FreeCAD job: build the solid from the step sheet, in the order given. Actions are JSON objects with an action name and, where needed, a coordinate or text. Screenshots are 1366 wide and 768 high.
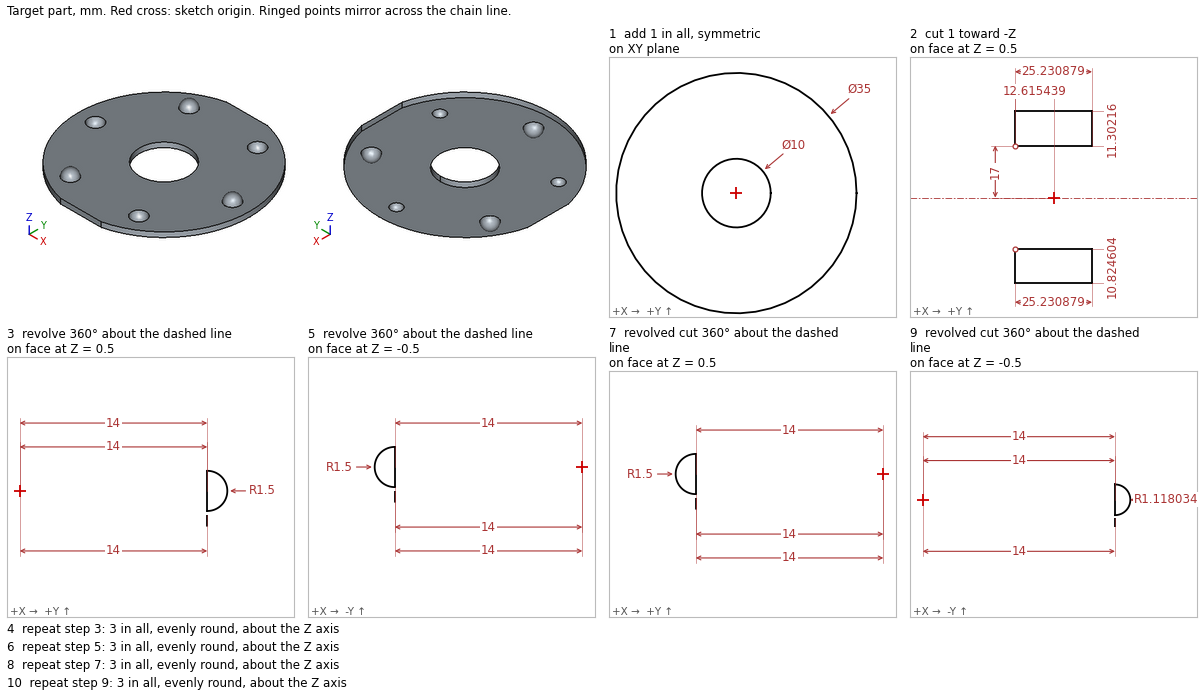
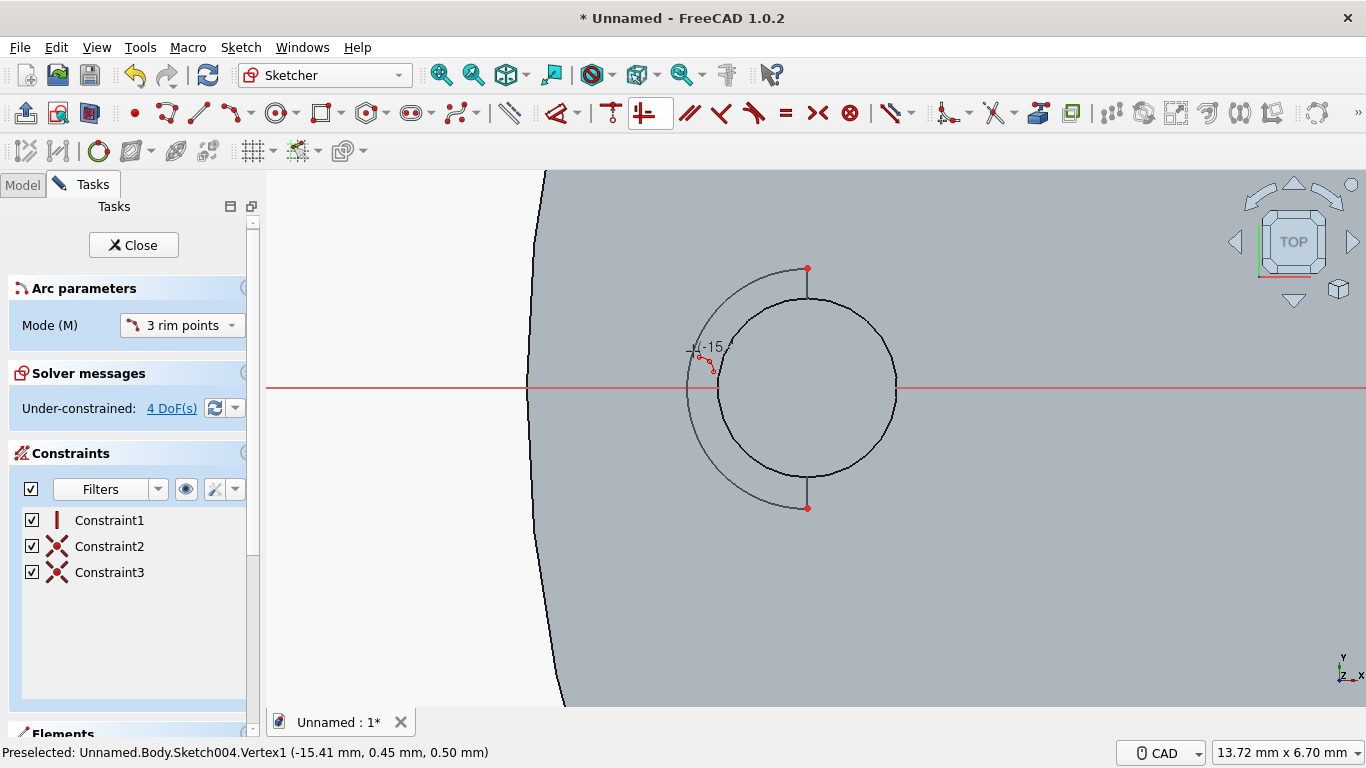
{"action": "key", "text": "g l"}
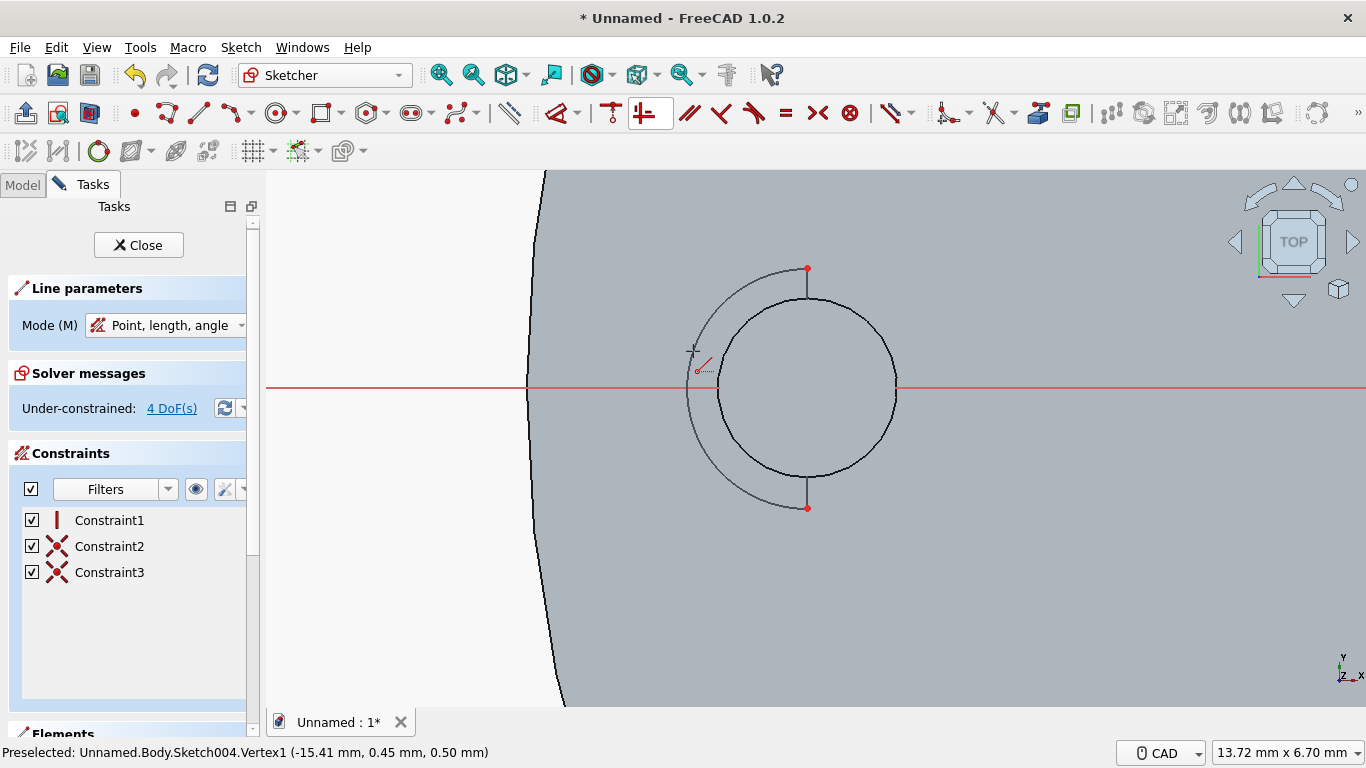
{"action": "left_click", "coordinate": [807, 532]}
{"action": "left_click", "coordinate": [807, 604]}
{"action": "key", "text": "Escape"}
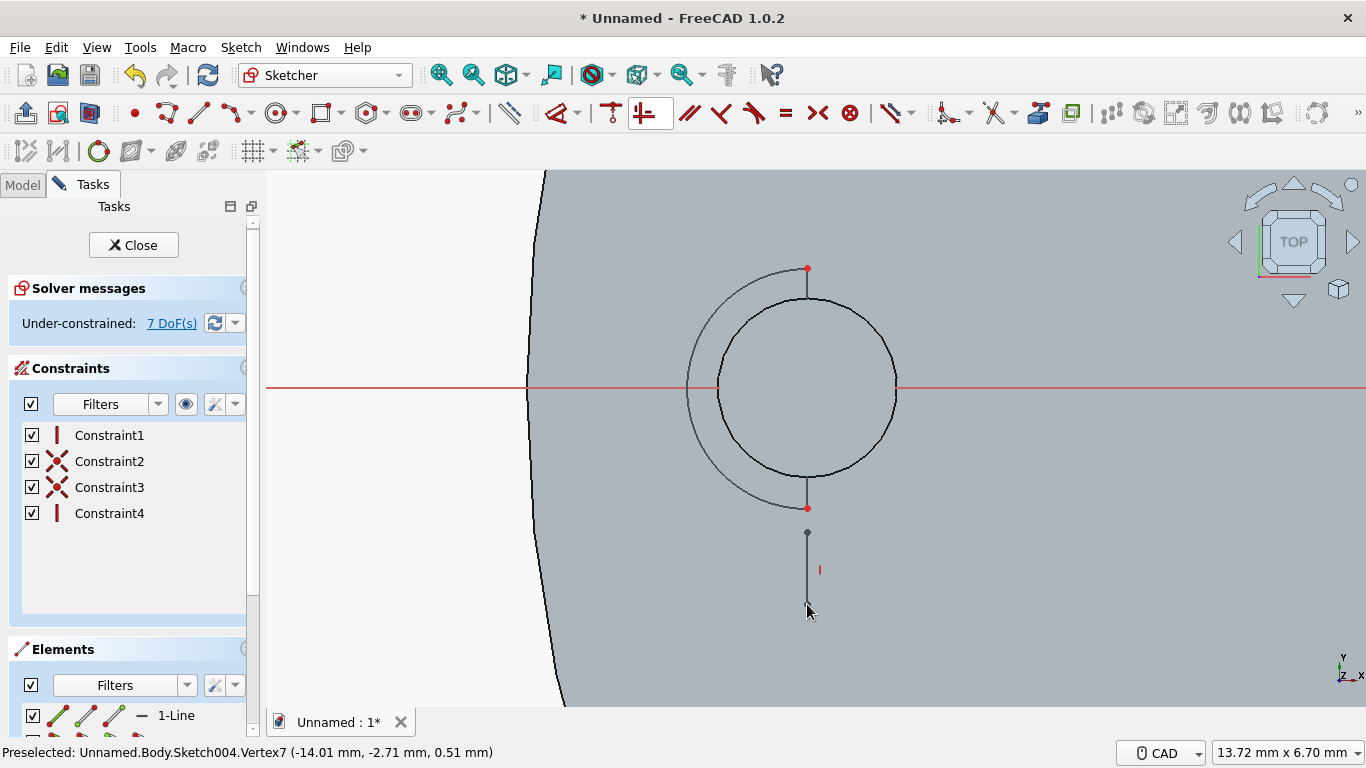
{"action": "left_click", "coordinate": [807, 555]}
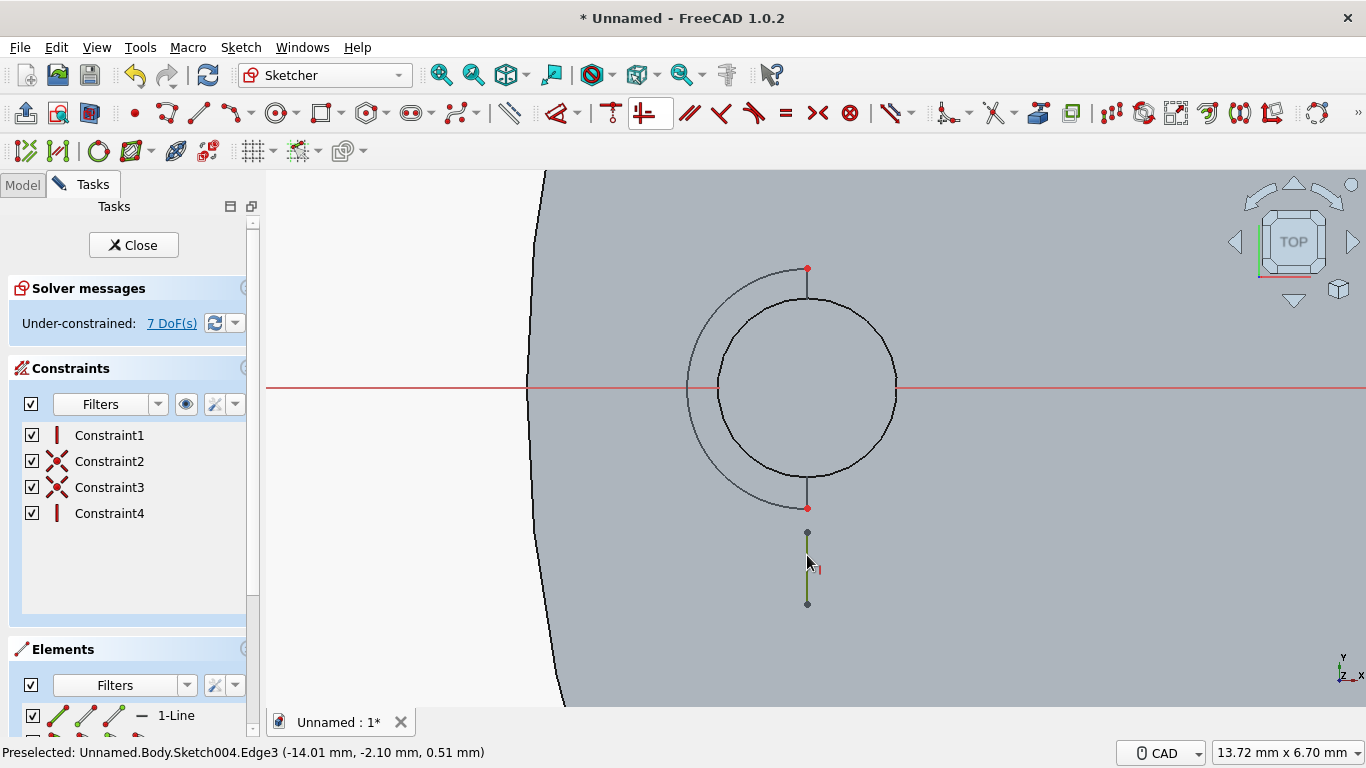
{"action": "key", "text": "g n"}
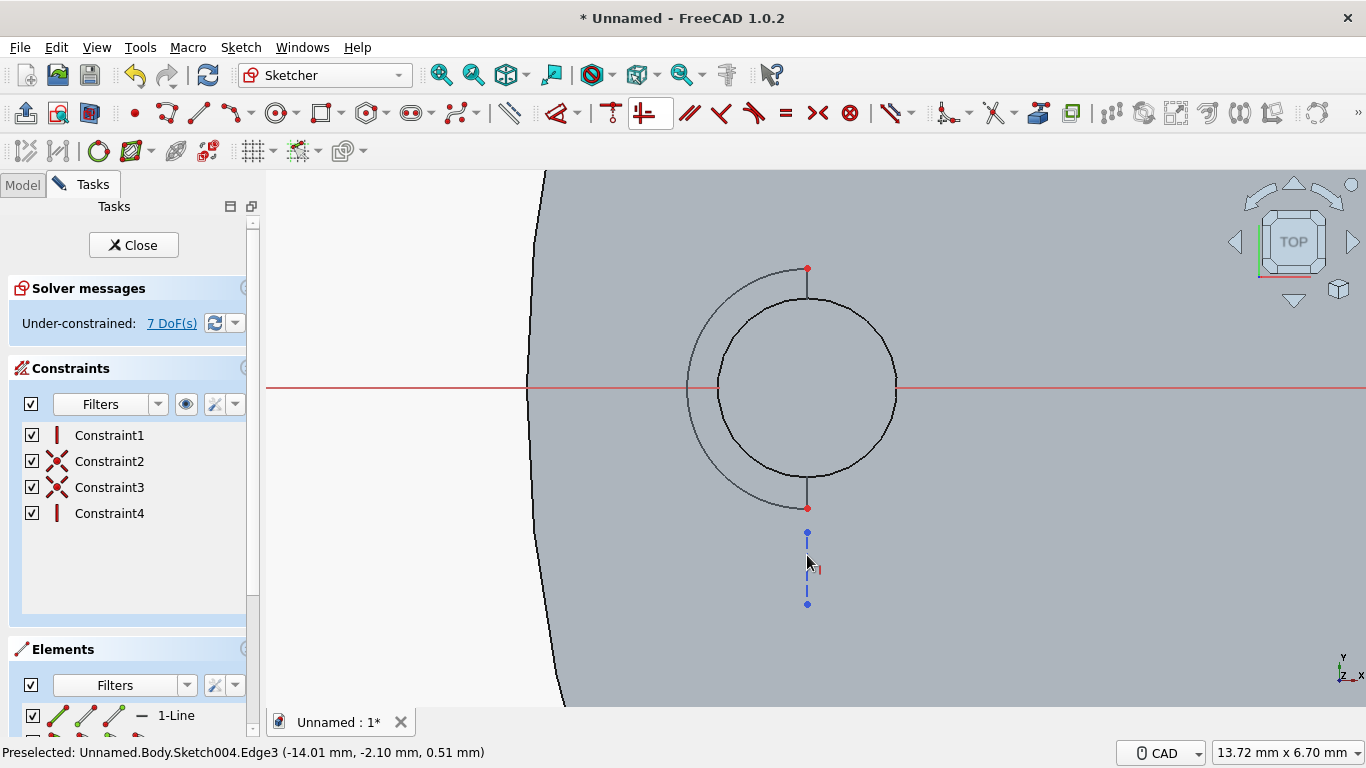
{"action": "left_click", "coordinate": [807, 389]}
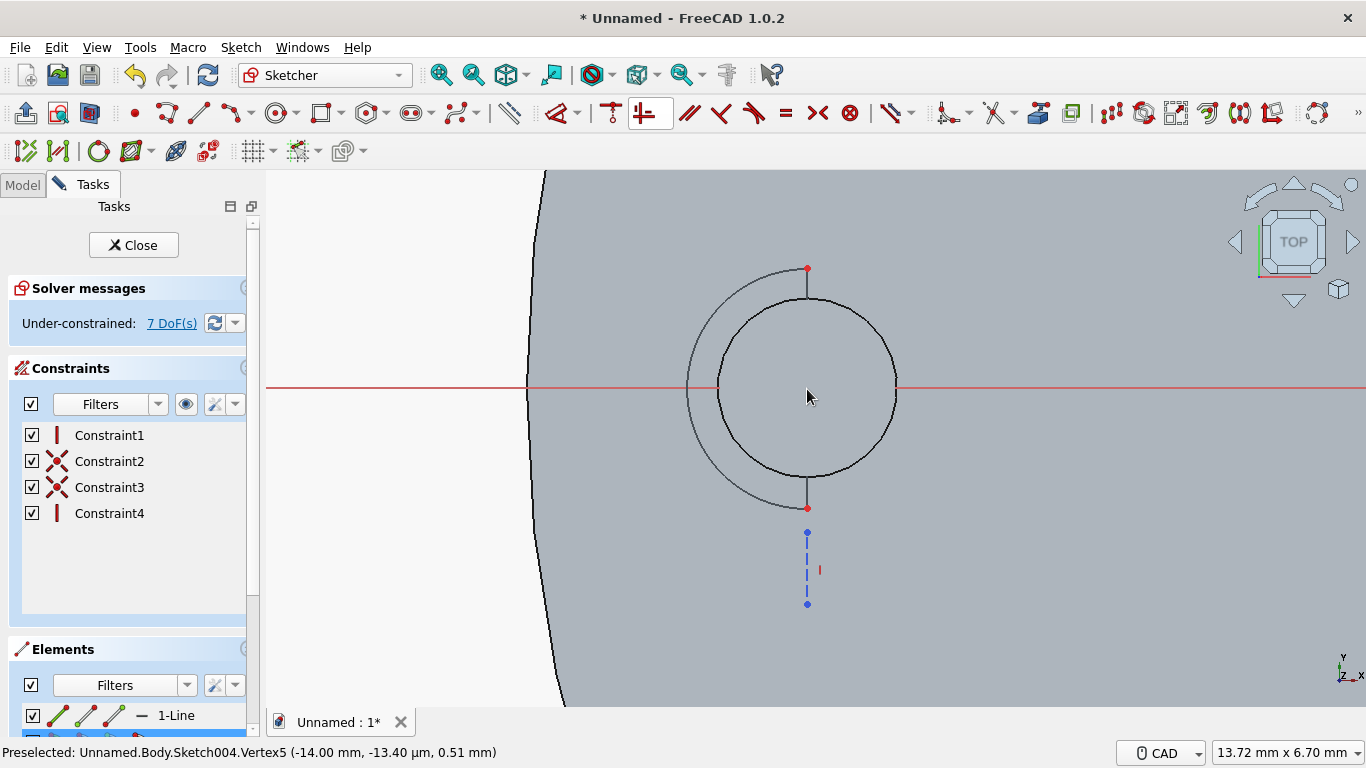
{"action": "left_click", "coordinate": [359, 388]}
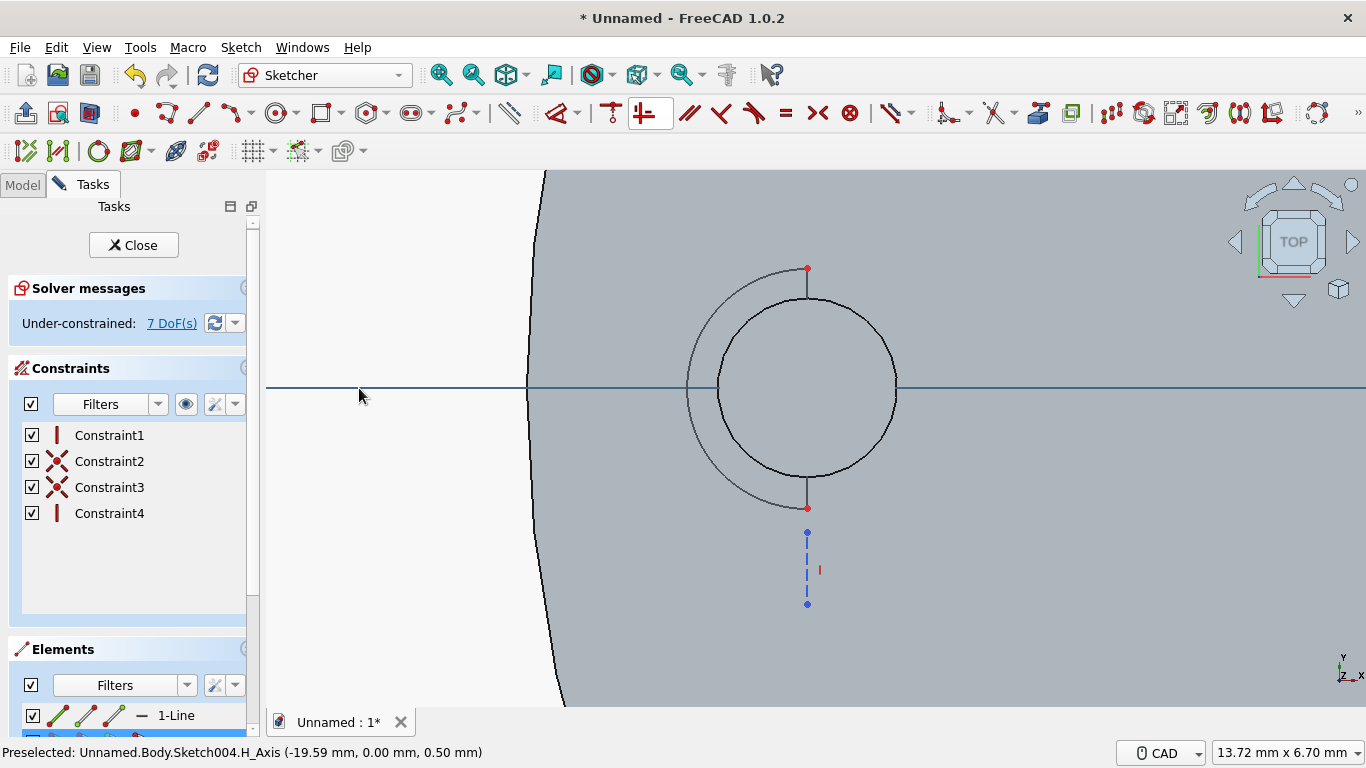
{"action": "left_click", "coordinate": [612, 114]}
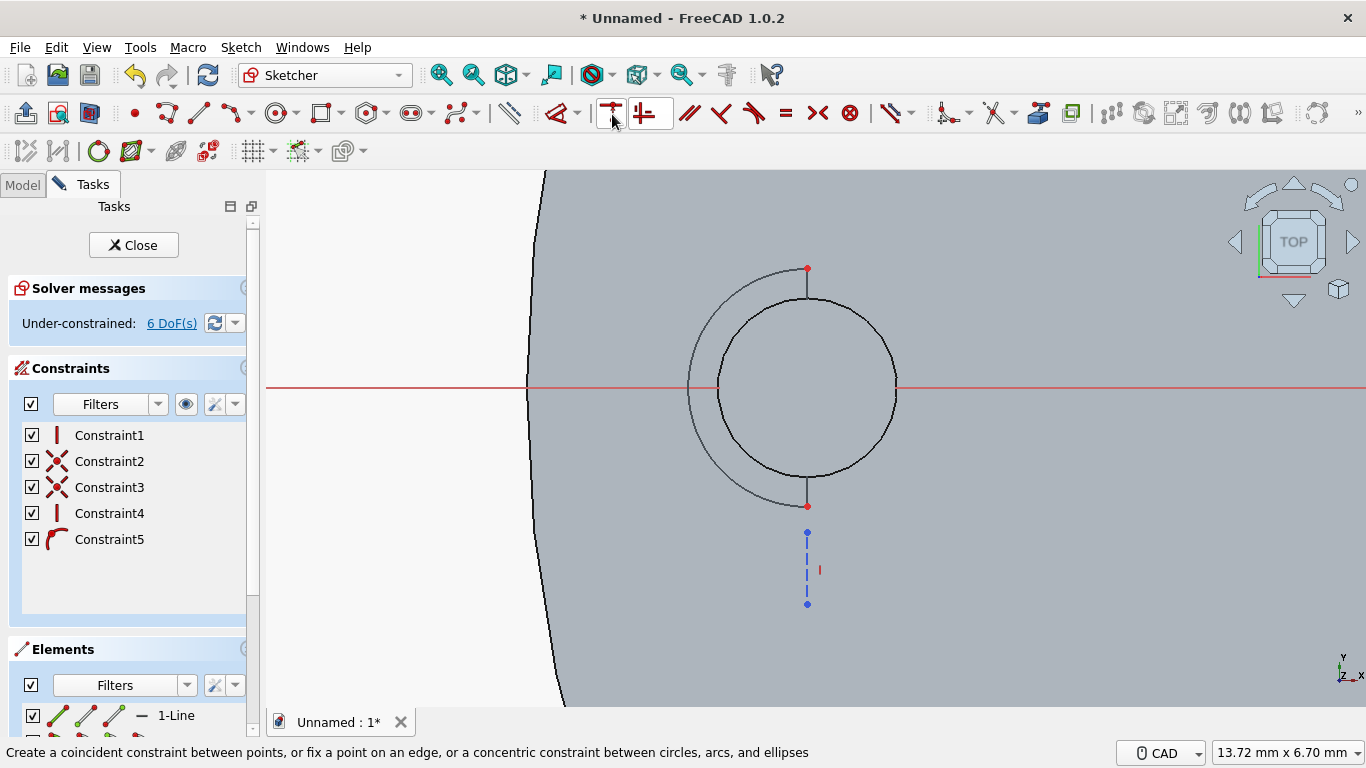
{"action": "key", "text": "d"}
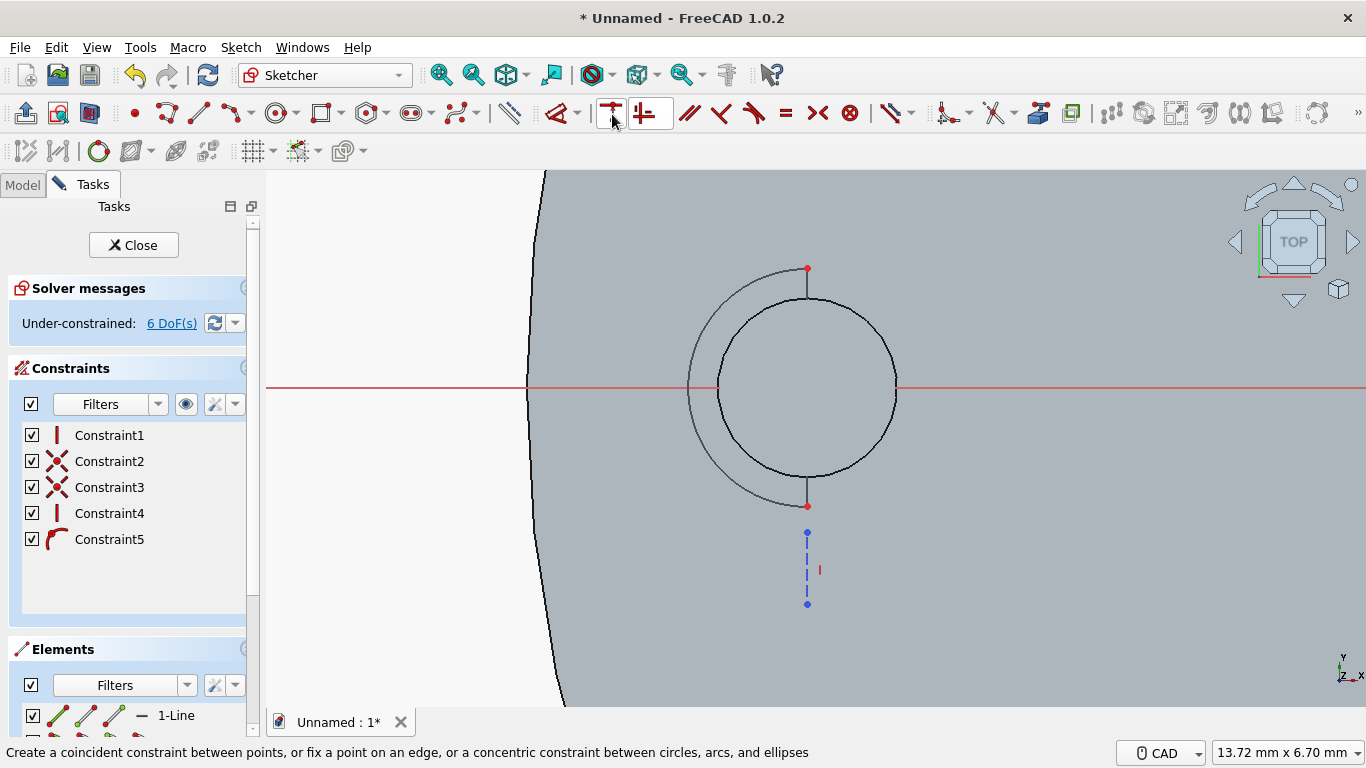
{"action": "left_click", "coordinate": [711, 318]}
{"action": "left_click", "coordinate": [685, 299]}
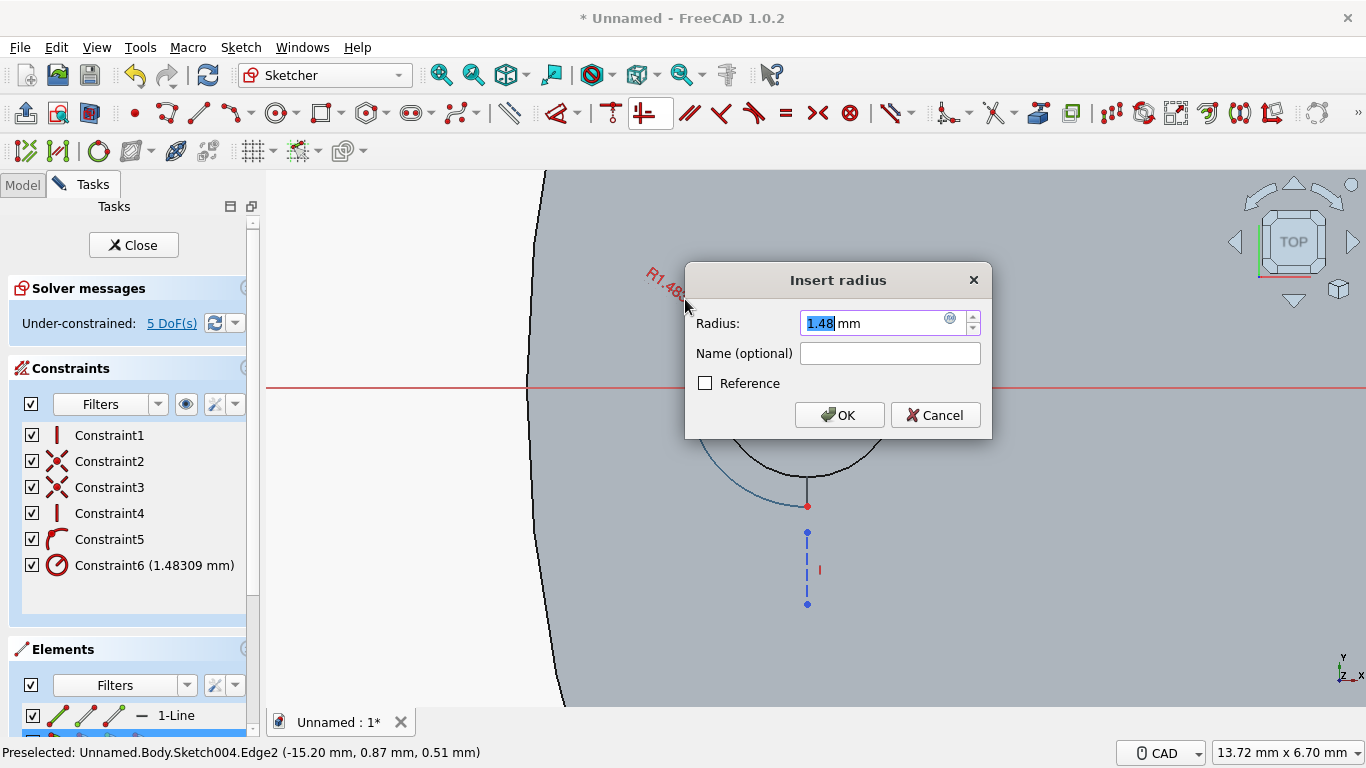
{"action": "type", "text": "1.5"}
{"action": "key", "text": "Return"}